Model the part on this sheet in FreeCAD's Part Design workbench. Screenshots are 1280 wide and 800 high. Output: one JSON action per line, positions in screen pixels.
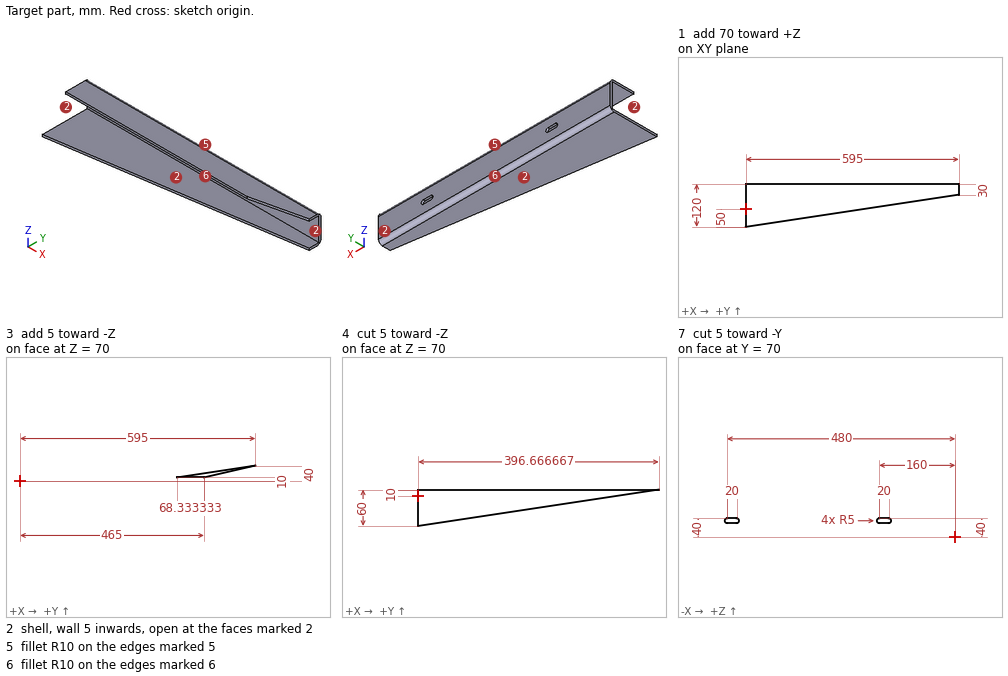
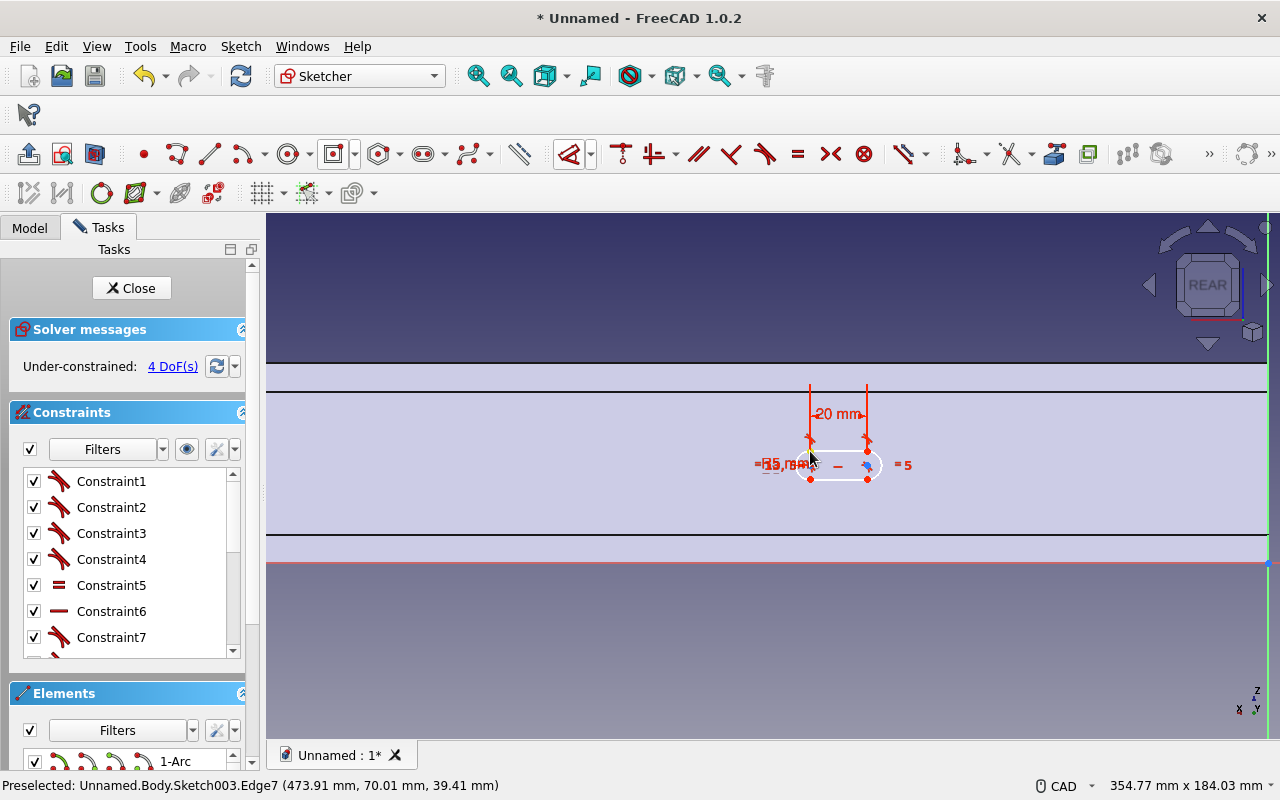
{"action": "left_click", "coordinate": [810, 451]}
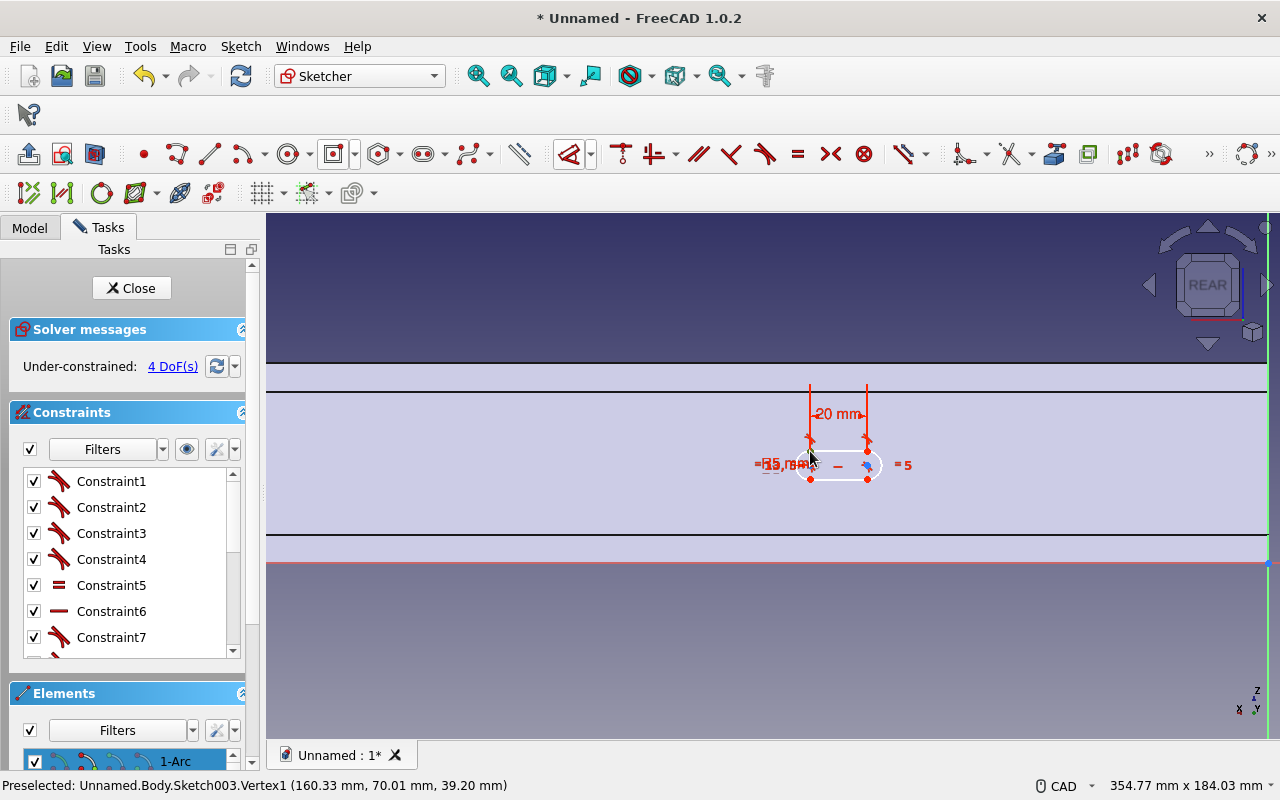
{"action": "left_click", "coordinate": [590, 154]}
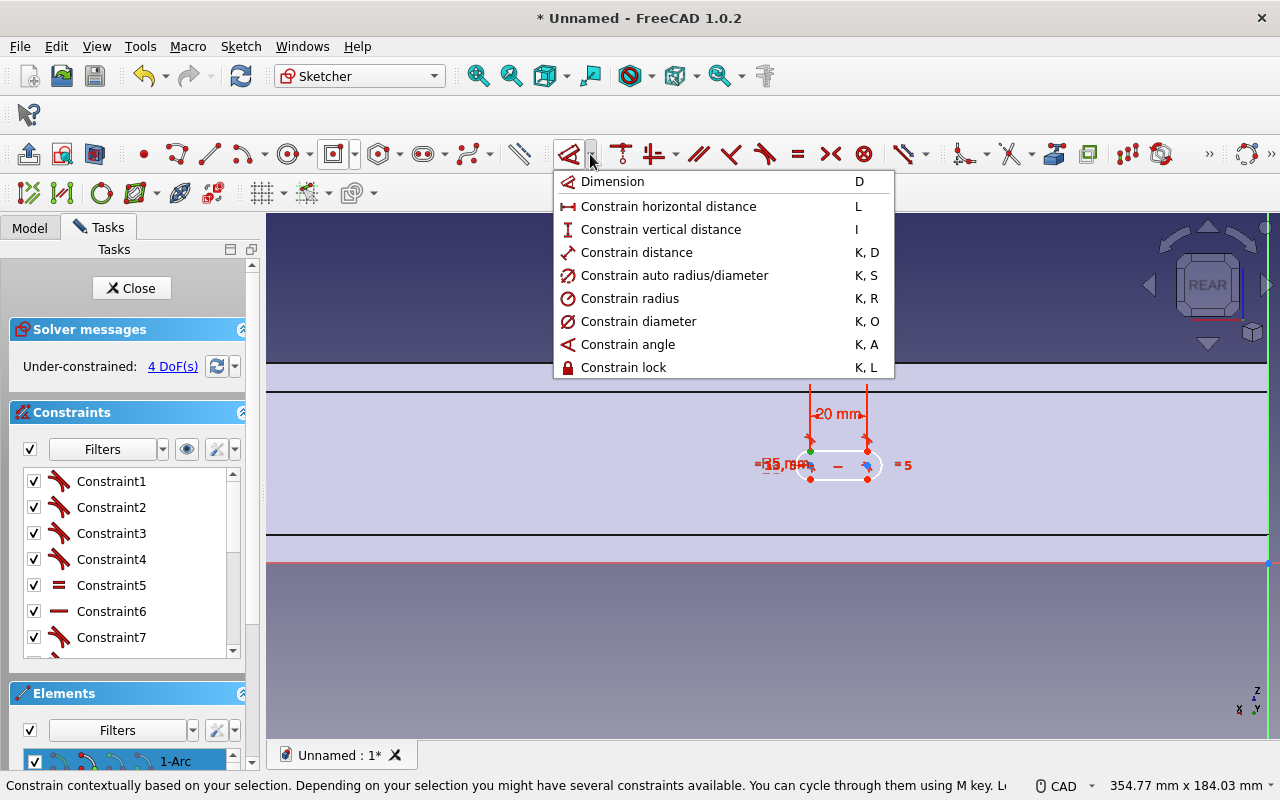
{"action": "left_click", "coordinate": [724, 230]}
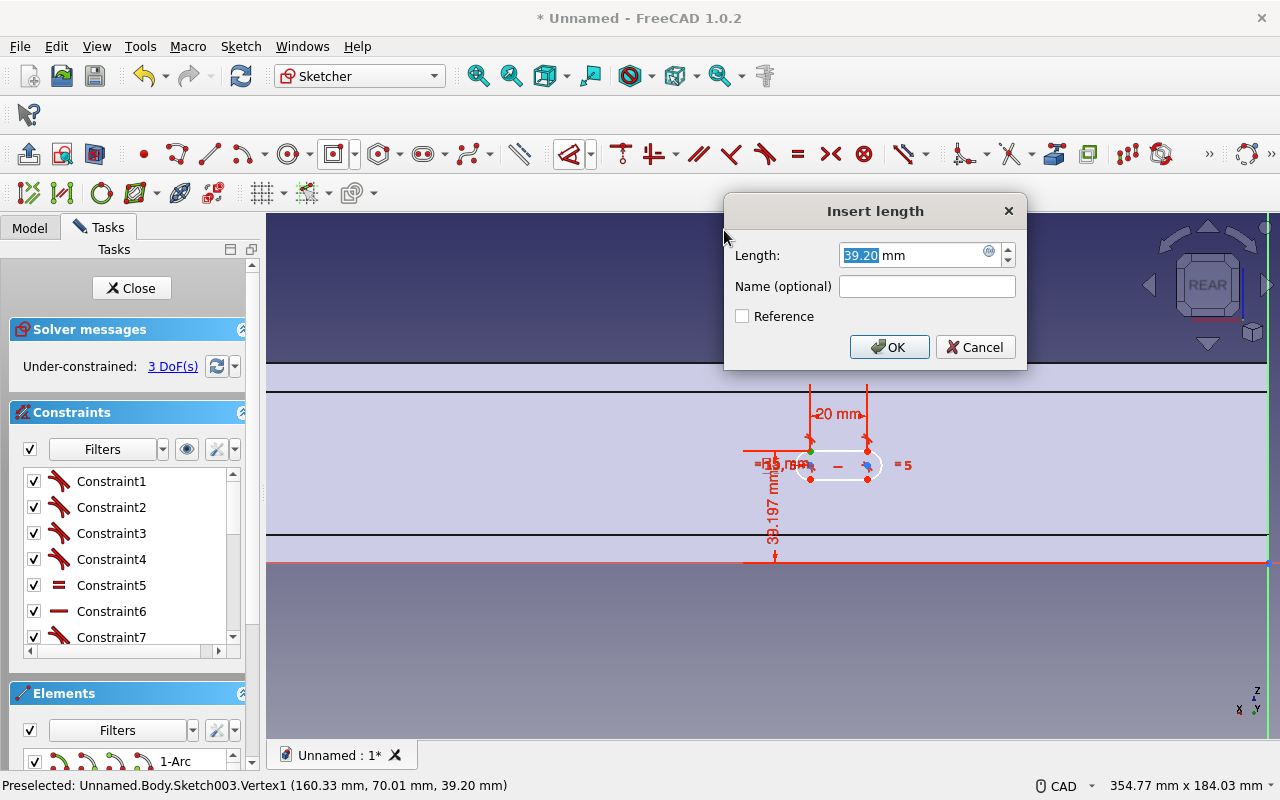
{"action": "type", "text": "40"}
{"action": "key", "text": "Return"}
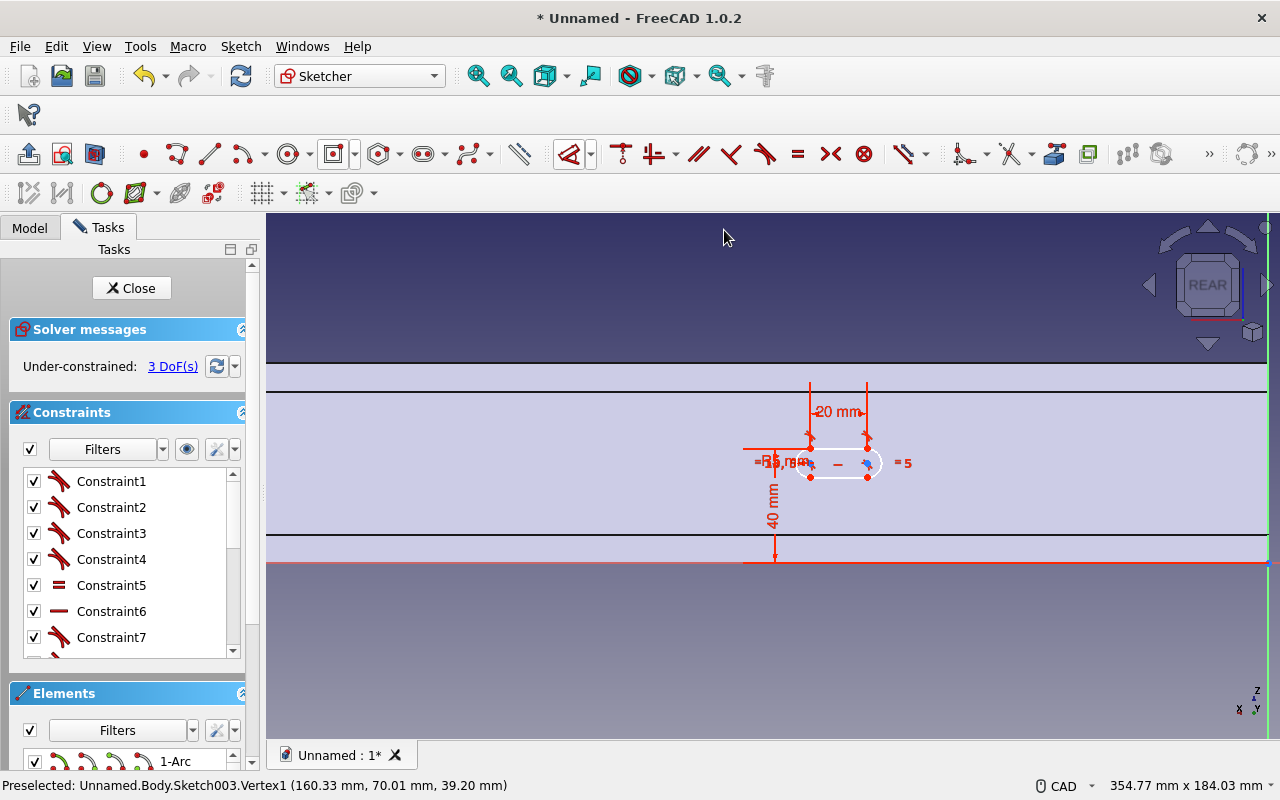
{"action": "scroll", "coordinate": [810, 451], "scroll_direction": "down", "scroll_amount": 4}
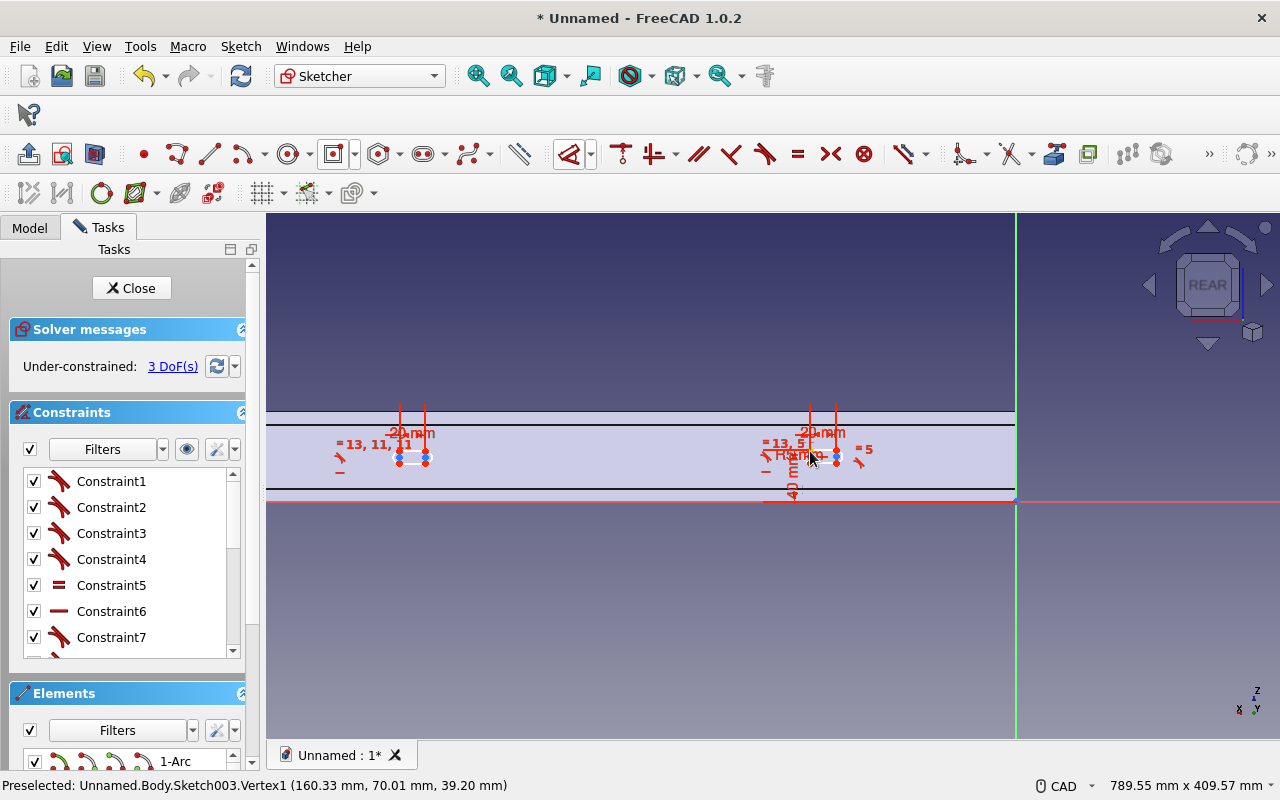
{"action": "scroll", "coordinate": [400, 451], "scroll_direction": "up", "scroll_amount": 4}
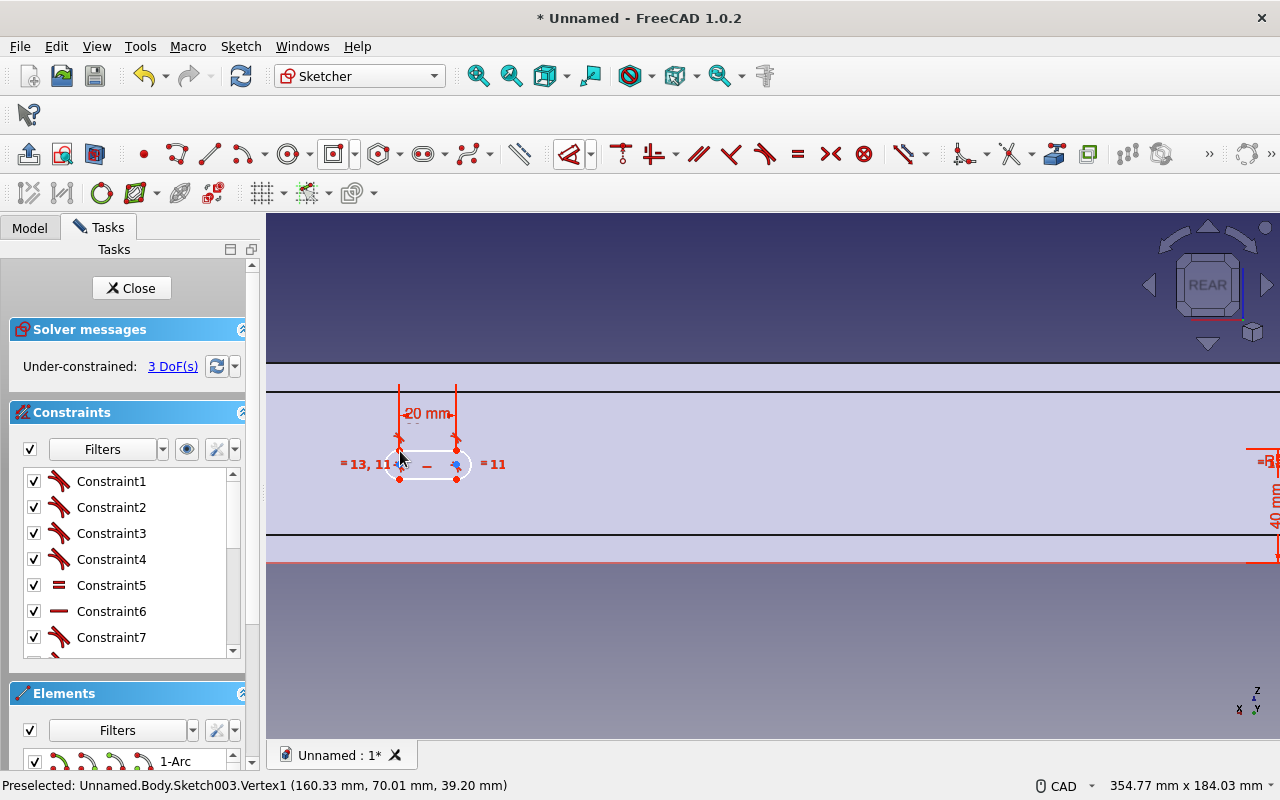
{"action": "left_click", "coordinate": [399, 451]}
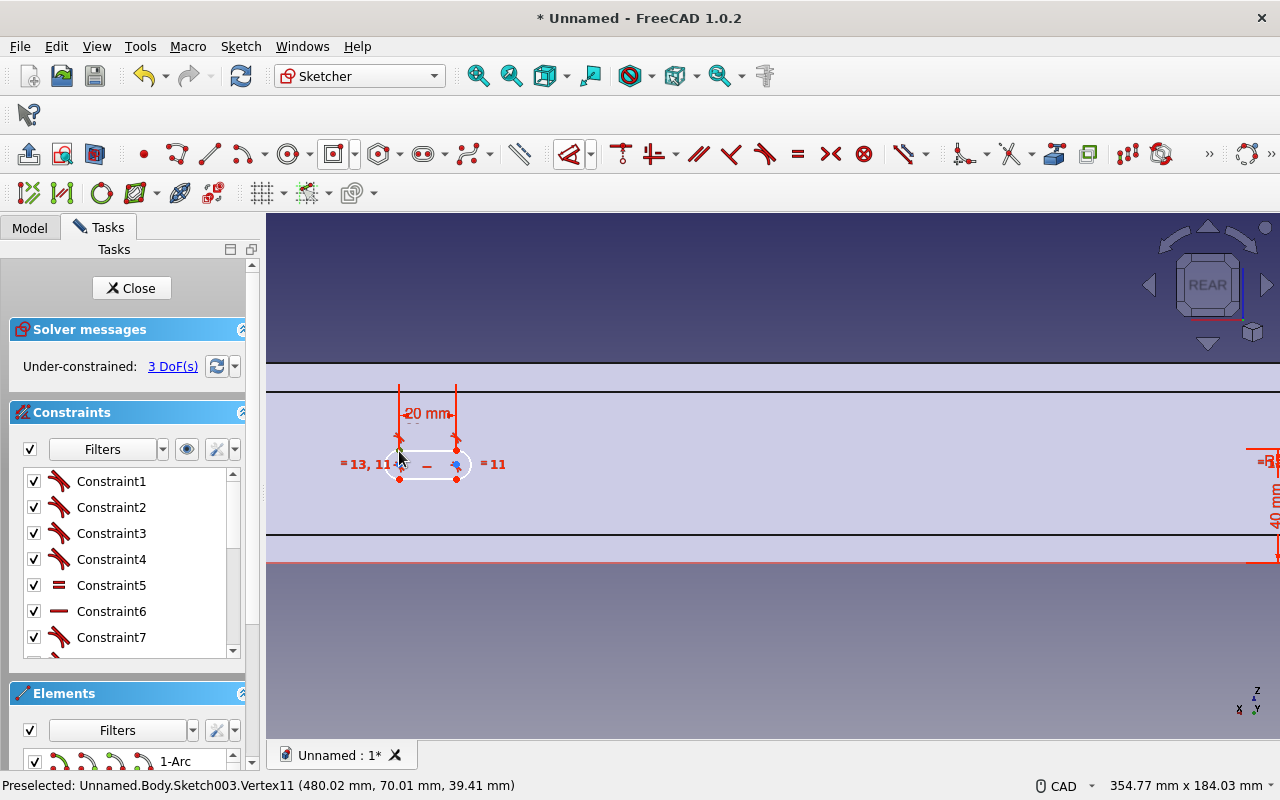
{"action": "key", "text": "i"}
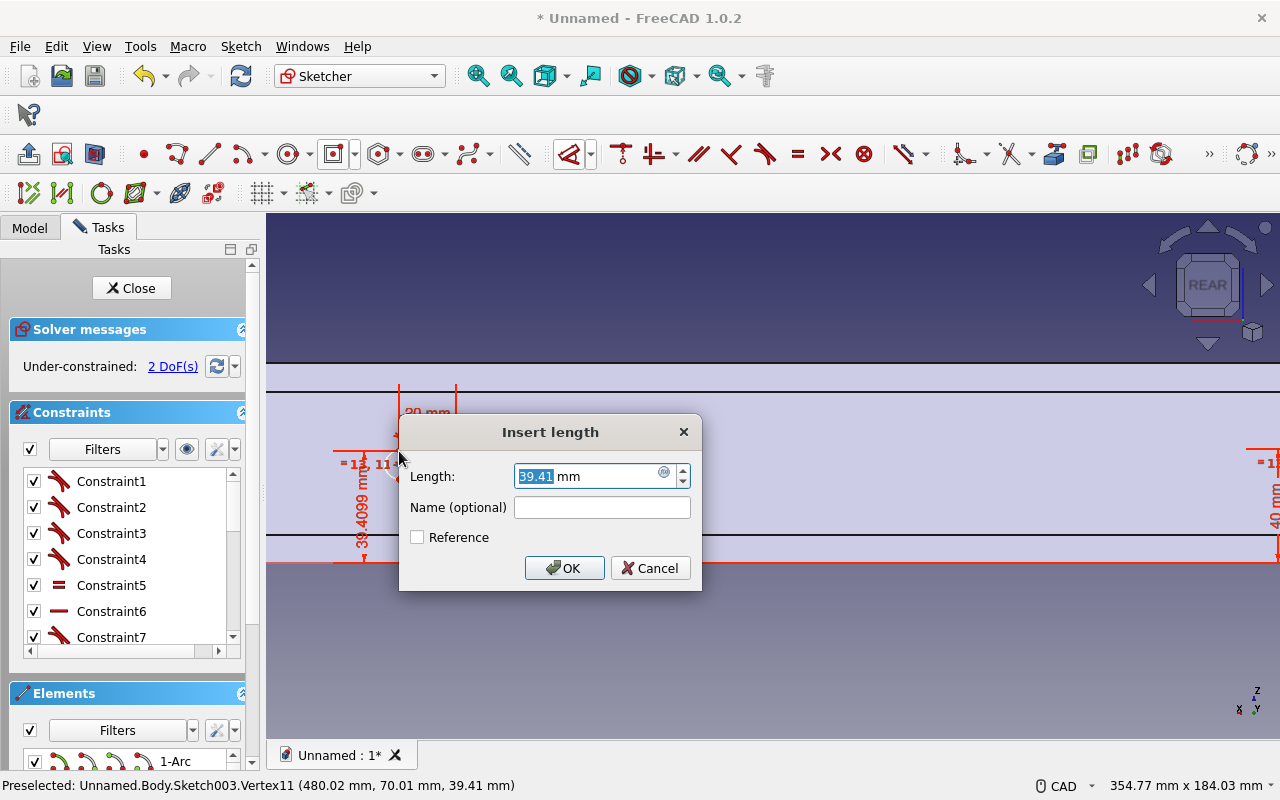
{"action": "type", "text": "40"}
{"action": "key", "text": "Return"}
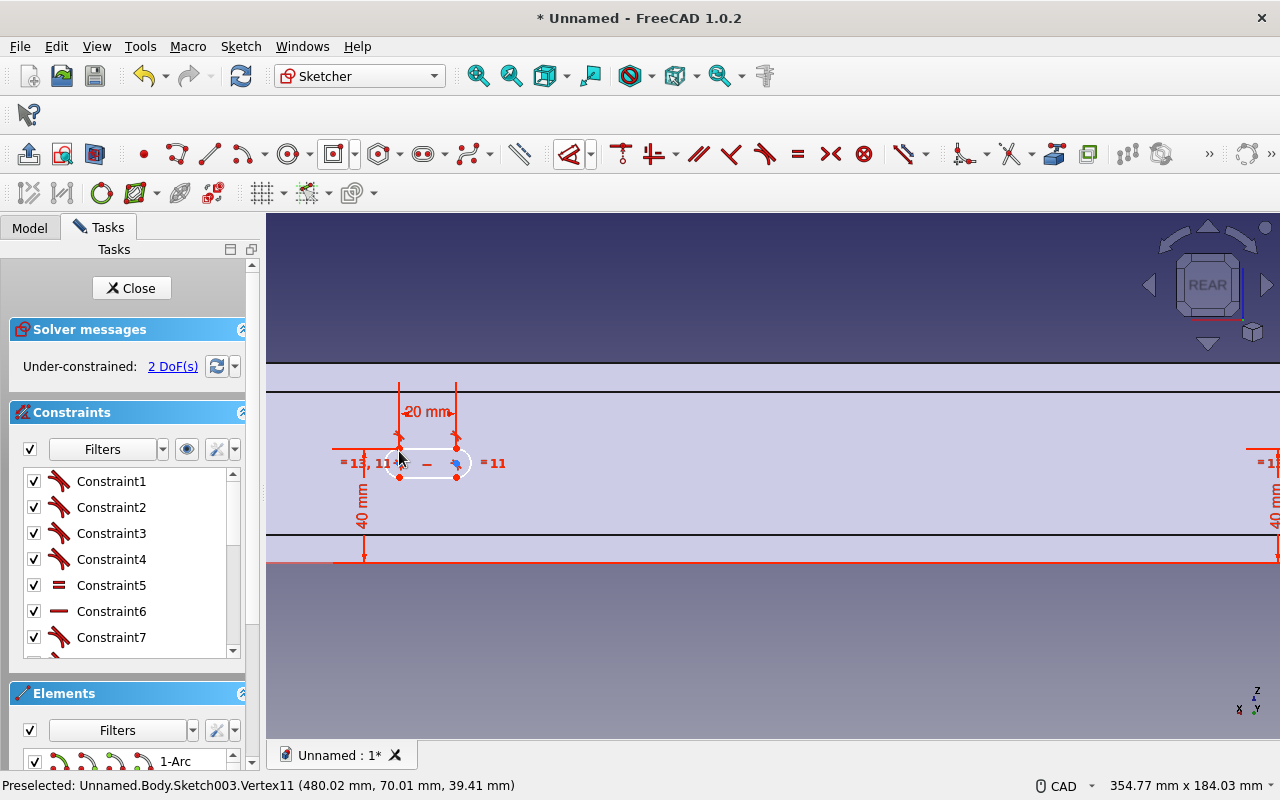
{"action": "scroll", "coordinate": [400, 451], "scroll_direction": "down", "scroll_amount": 4}